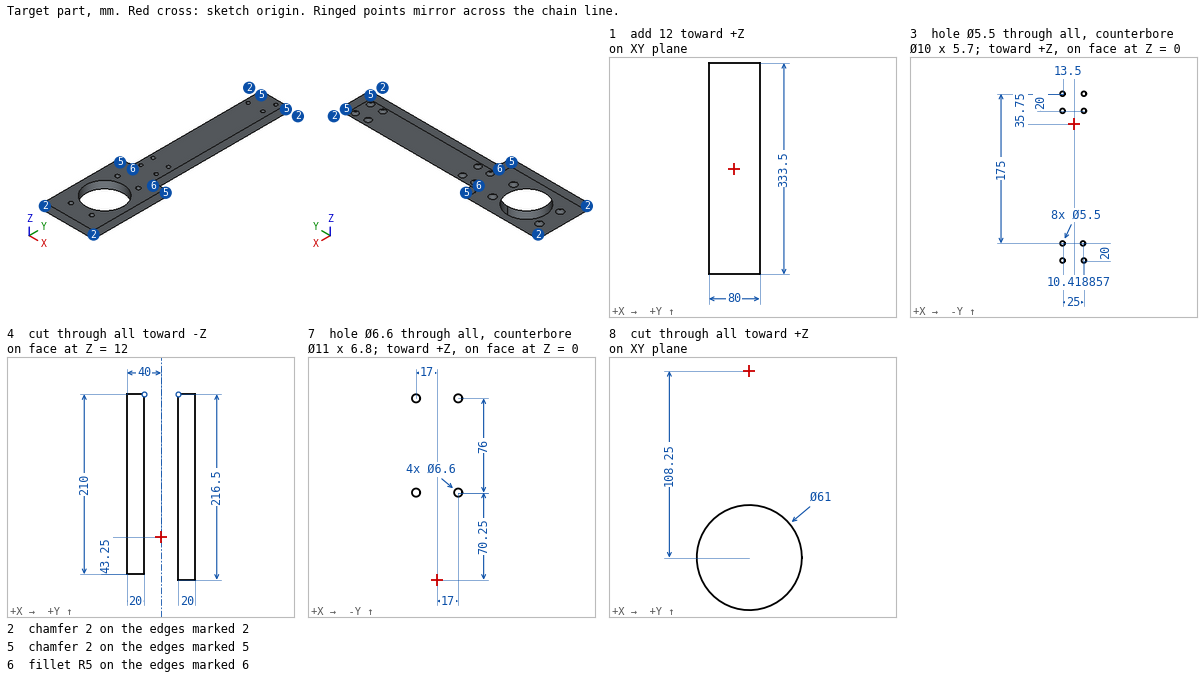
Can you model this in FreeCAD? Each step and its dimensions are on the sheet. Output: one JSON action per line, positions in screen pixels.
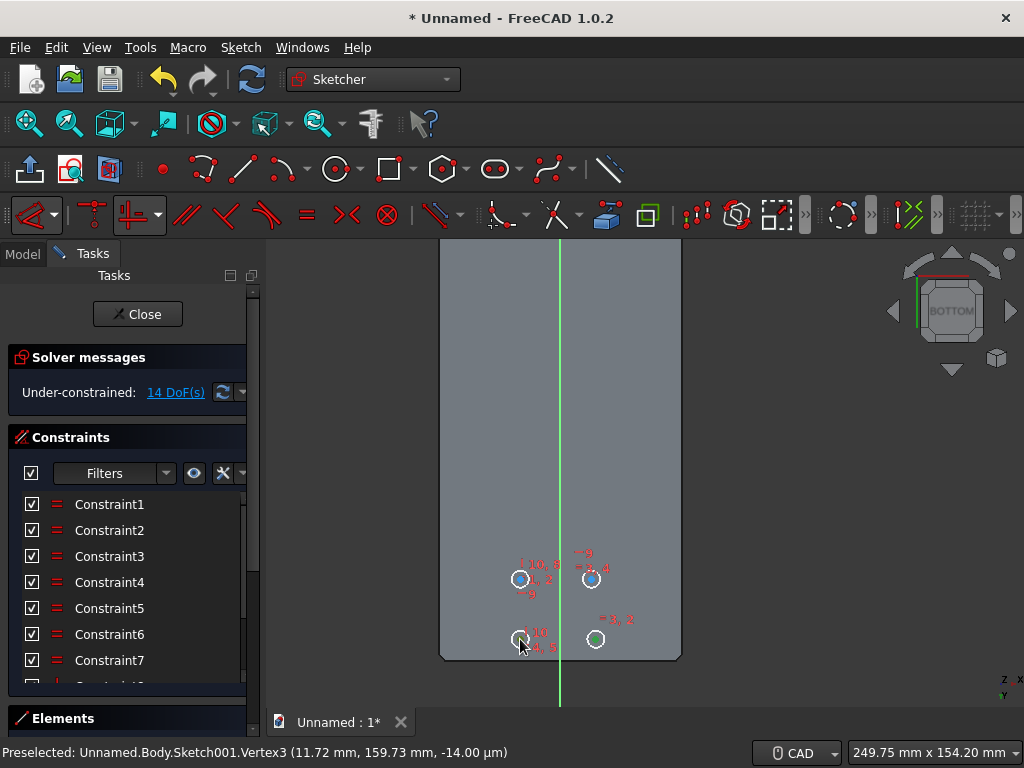
{"action": "key", "text": "h"}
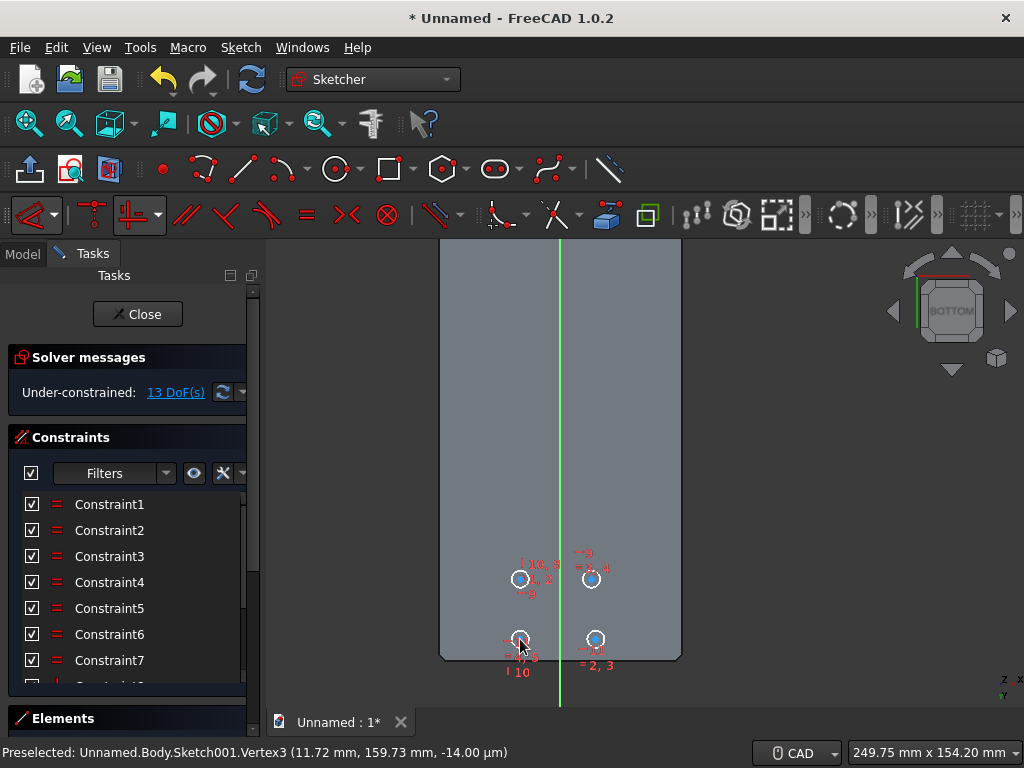
{"action": "left_click", "coordinate": [596, 639]}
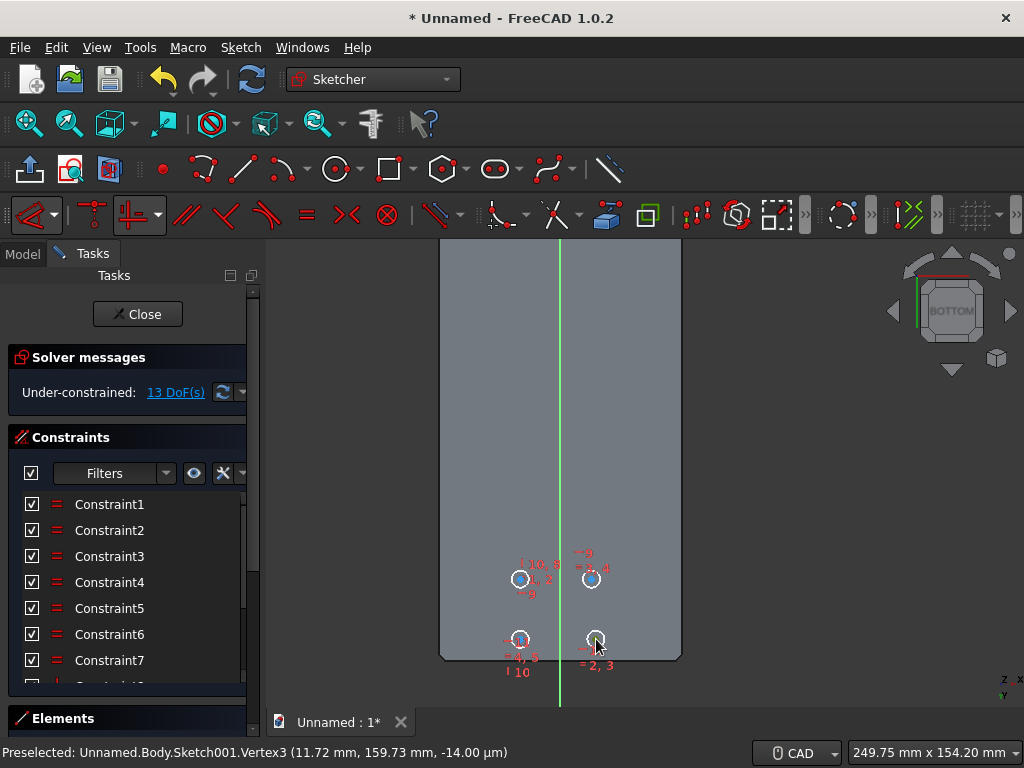
{"action": "scroll", "coordinate": [592, 580], "scroll_direction": "down", "scroll_amount": 4}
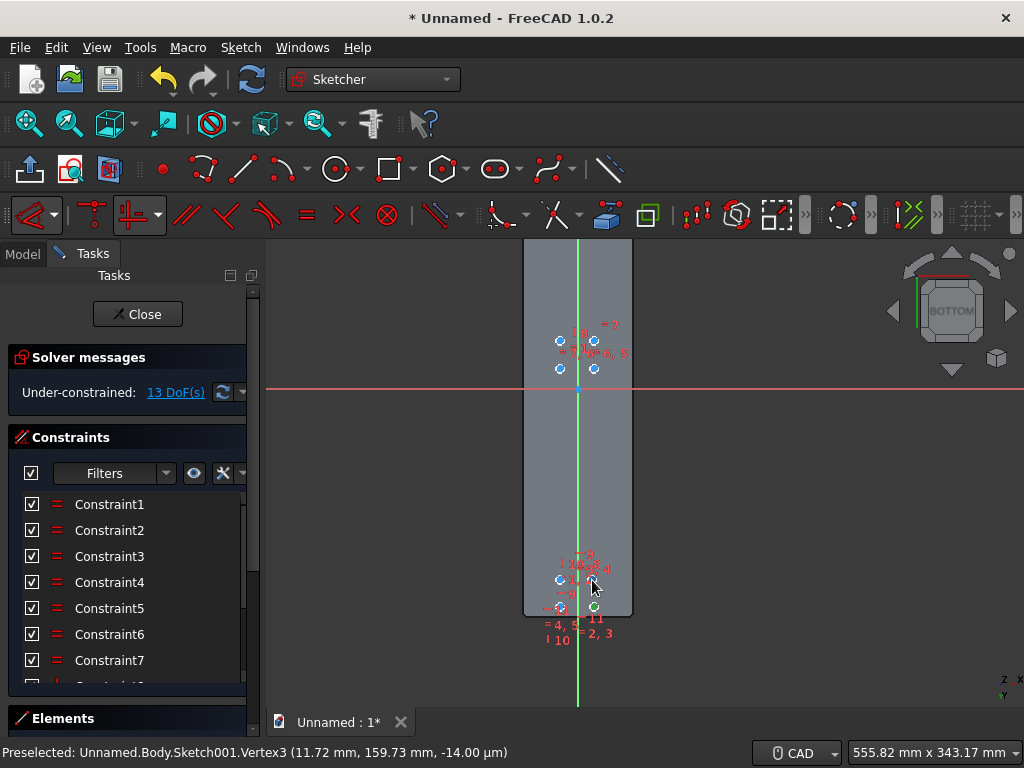
{"action": "left_click", "coordinate": [594, 369]}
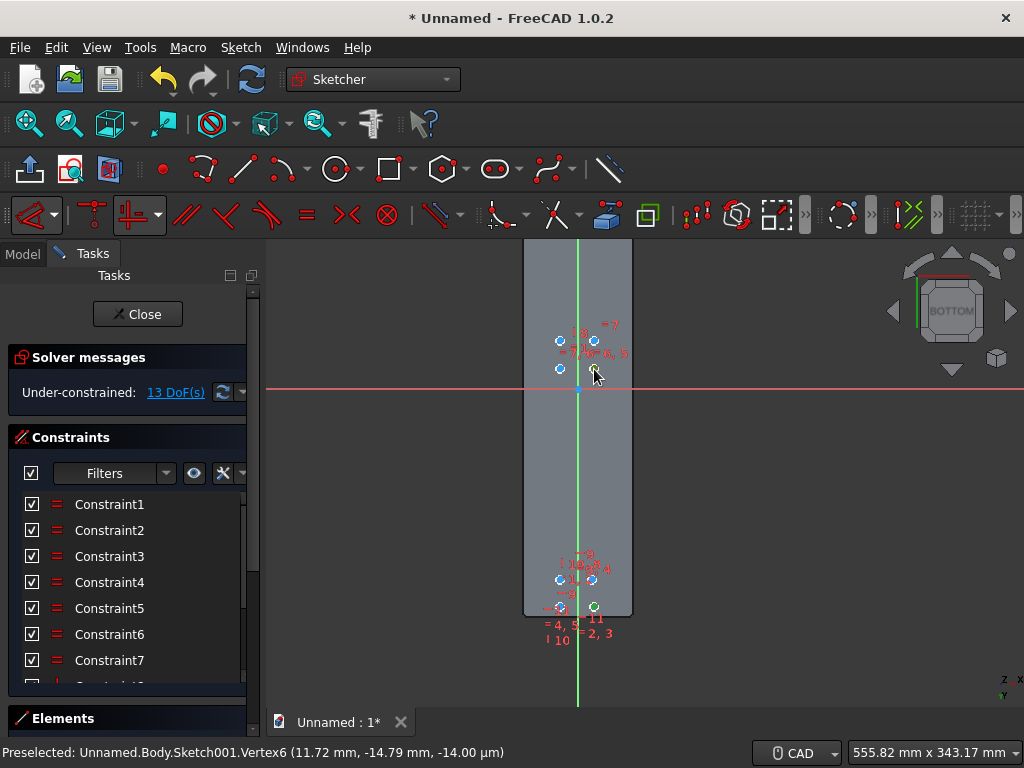
{"action": "left_click", "coordinate": [160, 216]}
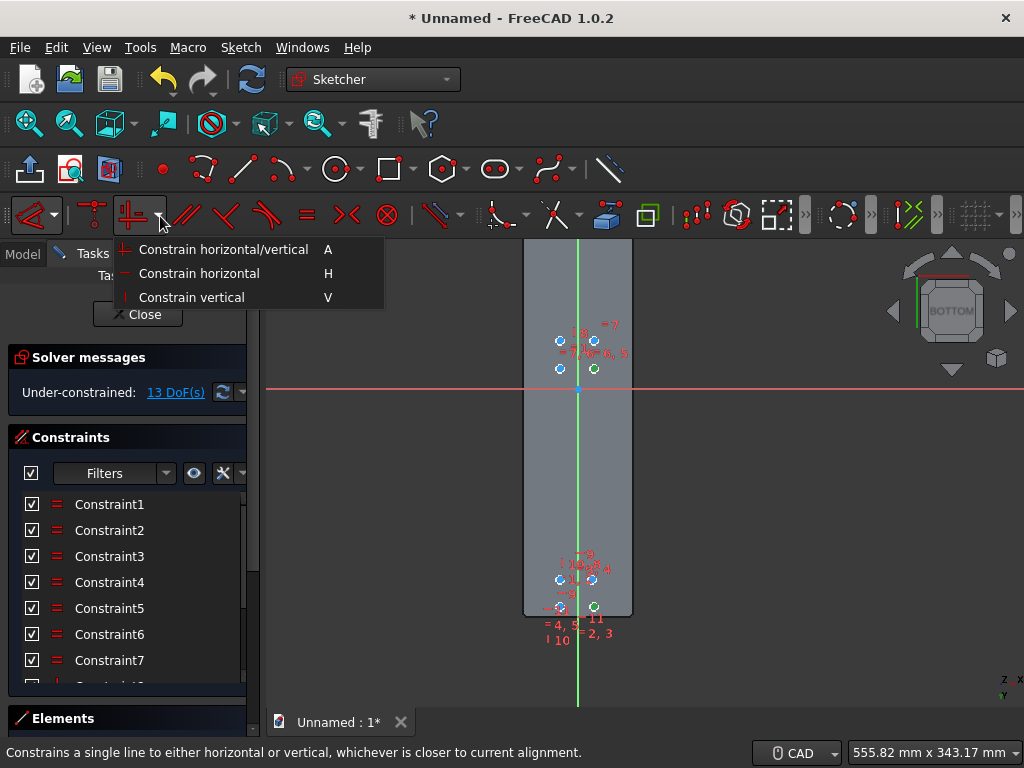
{"action": "left_click", "coordinate": [249, 297]}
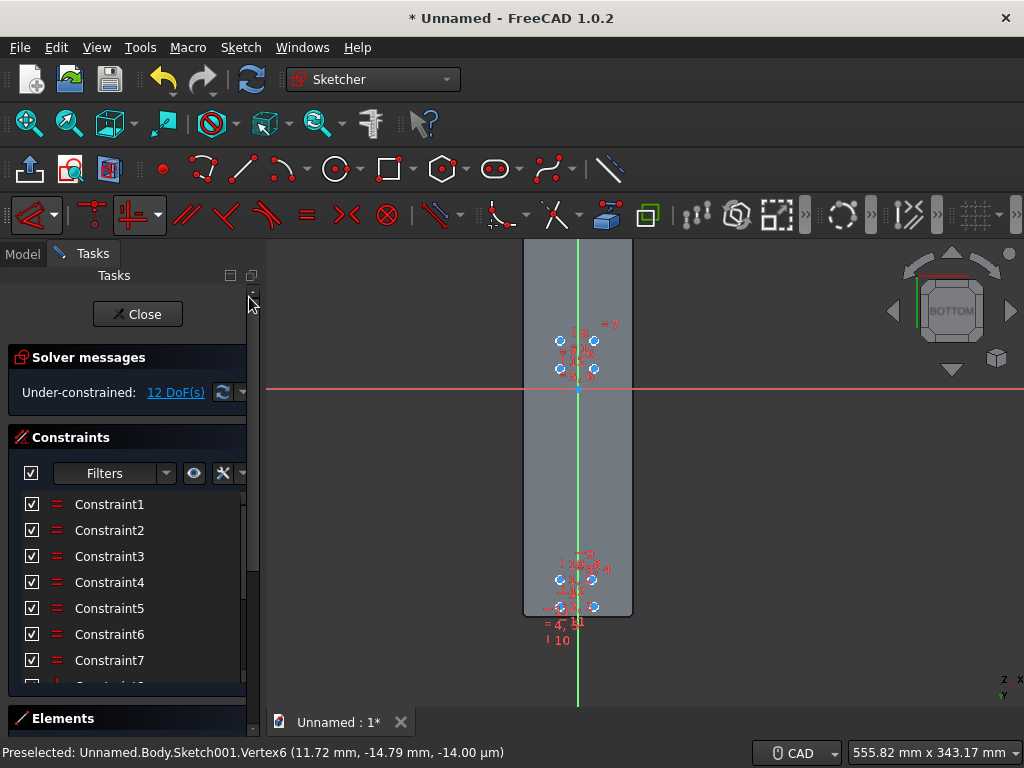
{"action": "left_click", "coordinate": [560, 341]}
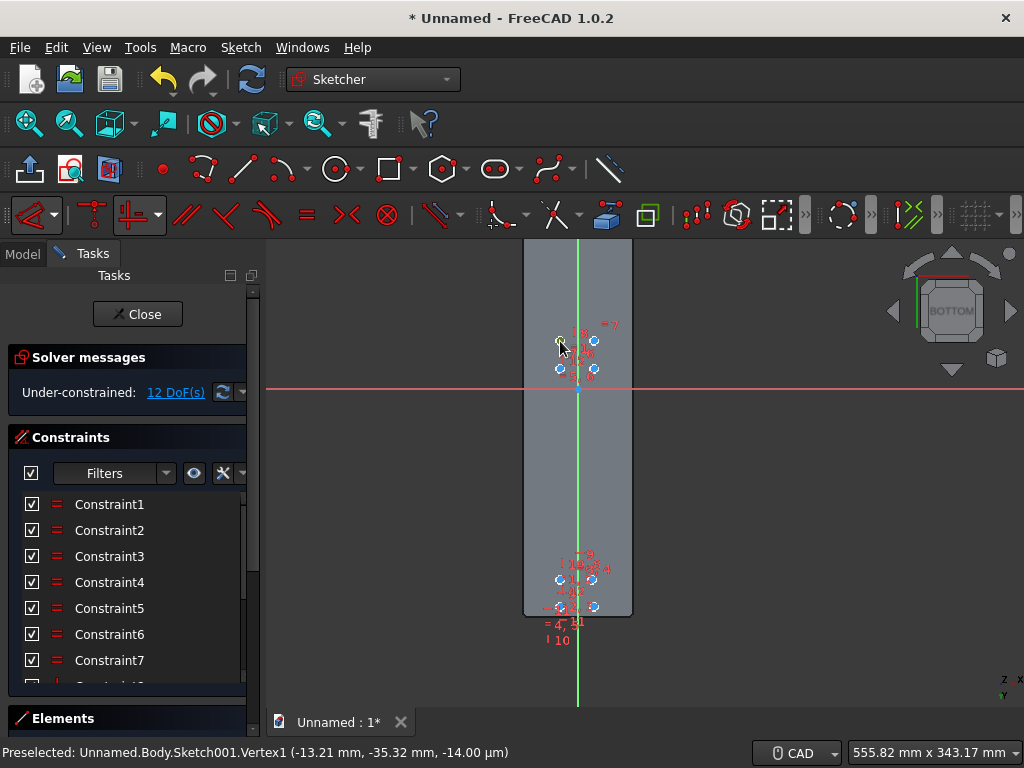
{"action": "scroll", "coordinate": [560, 369], "scroll_direction": "up", "scroll_amount": 4}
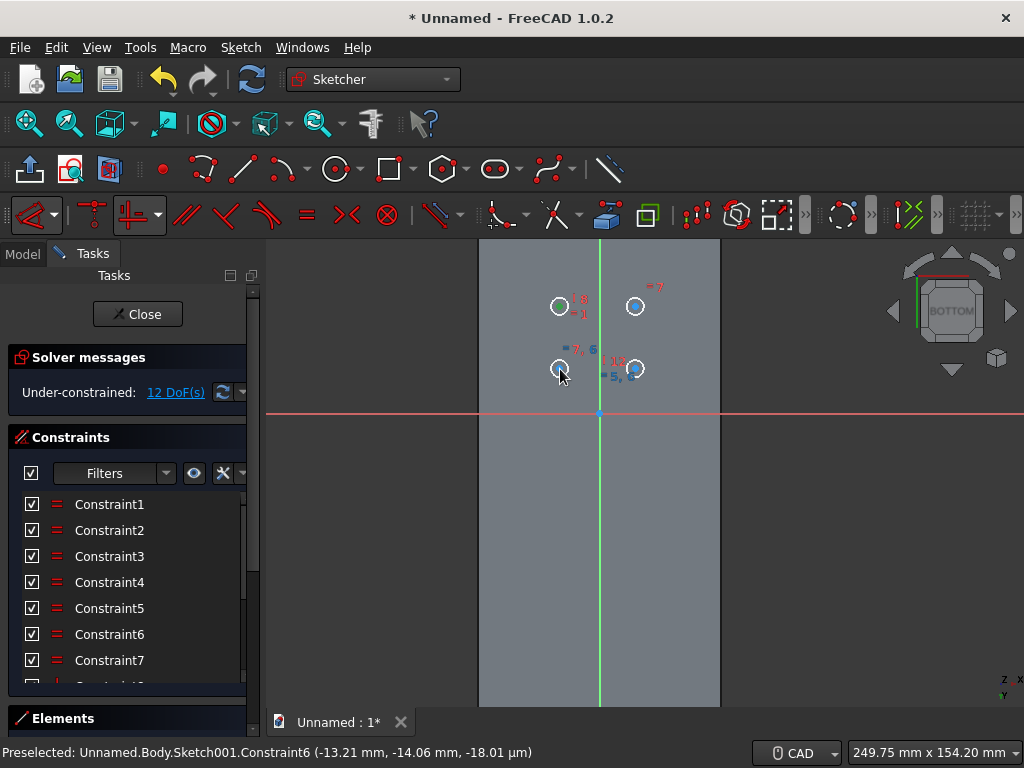
{"action": "left_click", "coordinate": [560, 369]}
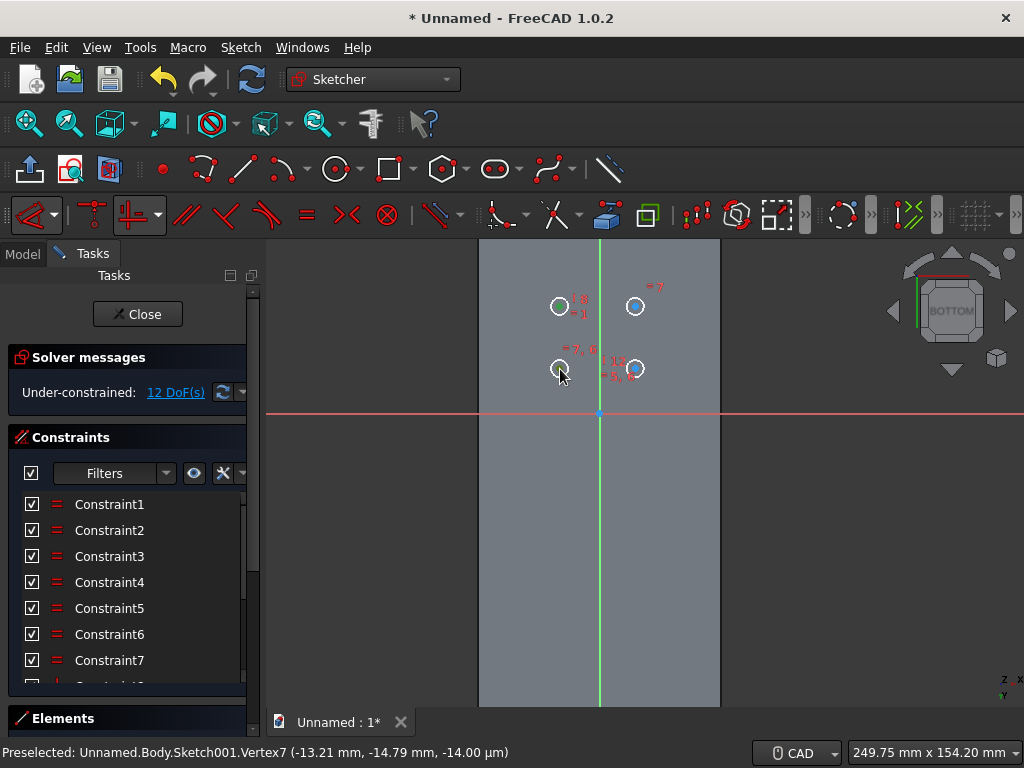
{"action": "left_click", "coordinate": [160, 216]}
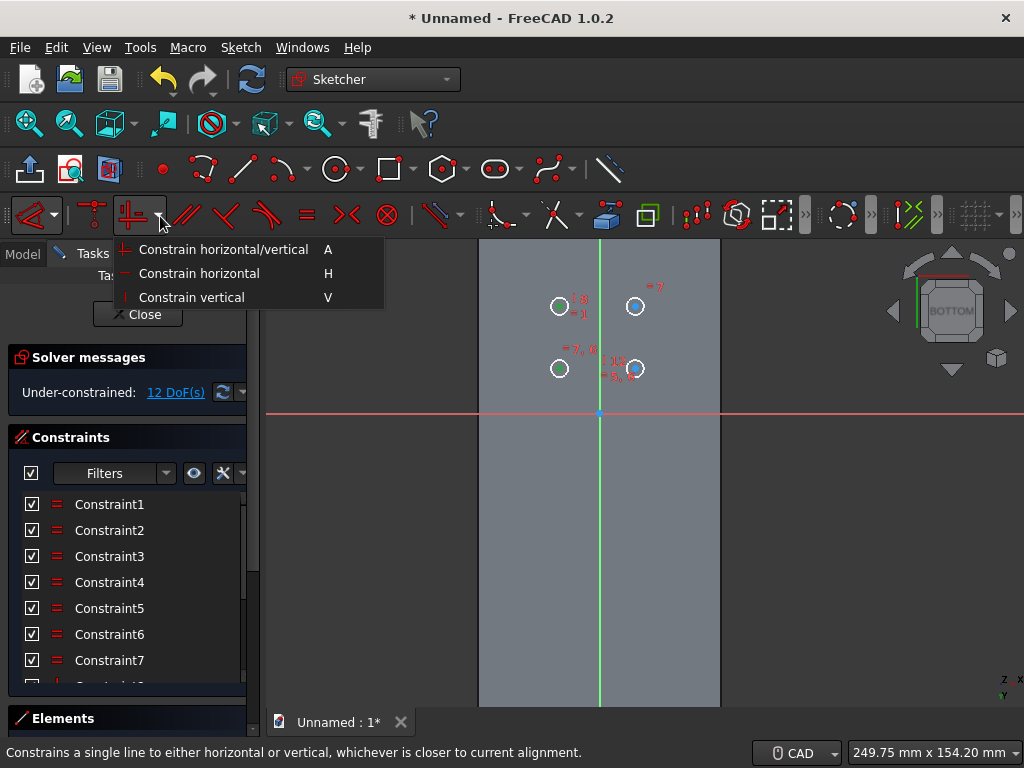
{"action": "left_click", "coordinate": [249, 297]}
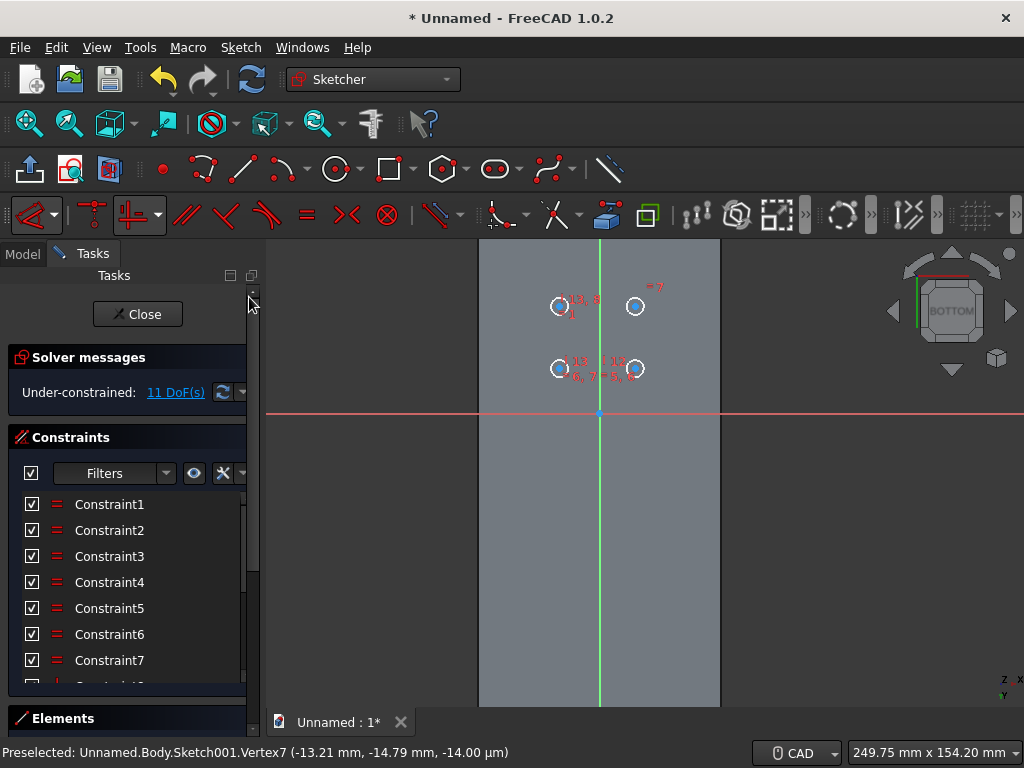
{"action": "left_click", "coordinate": [635, 369]}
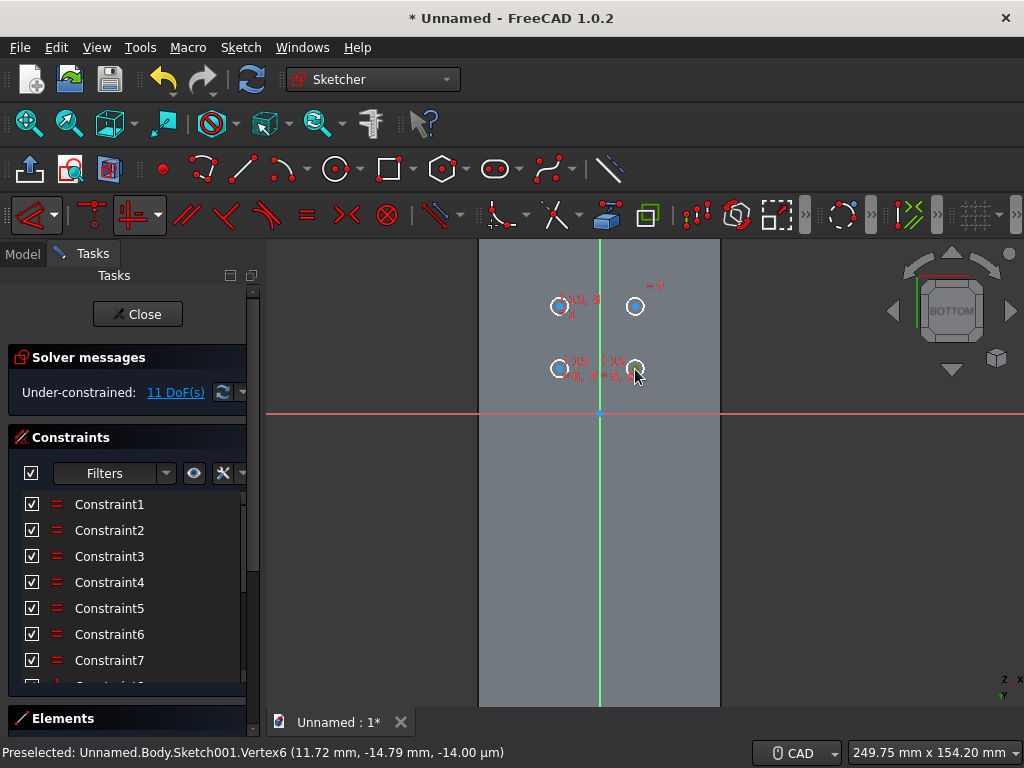
{"action": "left_click", "coordinate": [558, 371]}